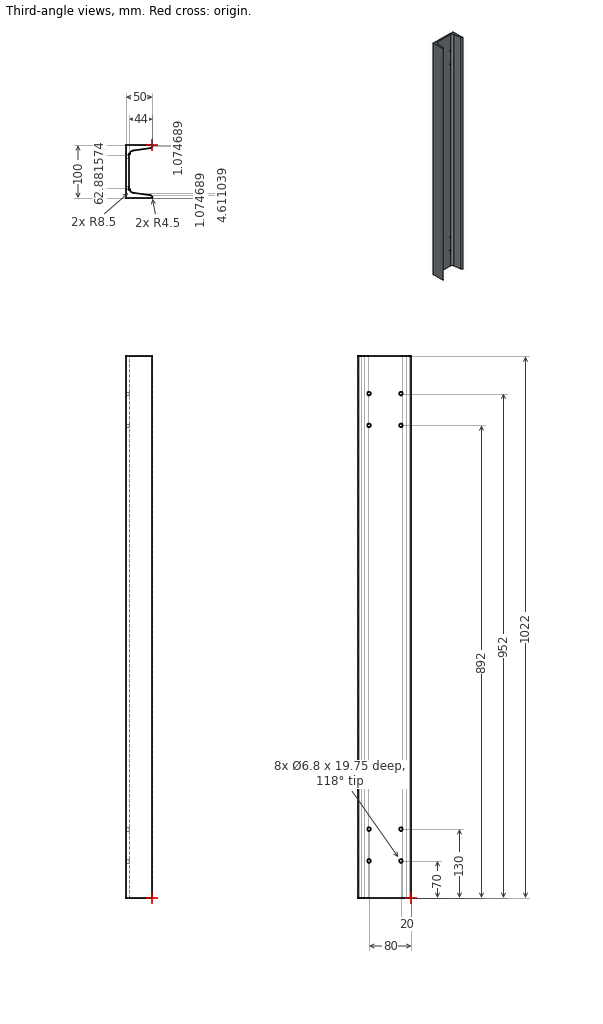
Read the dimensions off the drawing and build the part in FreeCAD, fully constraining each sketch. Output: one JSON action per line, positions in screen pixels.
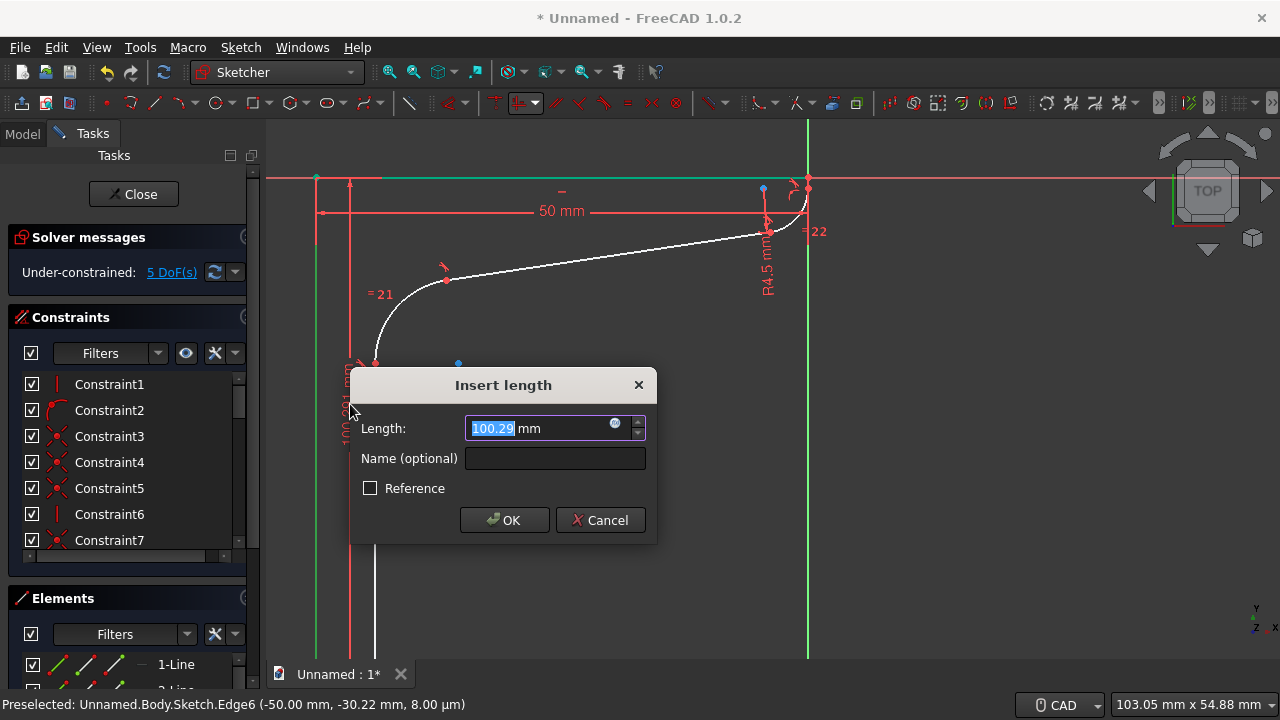
{"action": "type", "text": "100"}
{"action": "key", "text": "Return"}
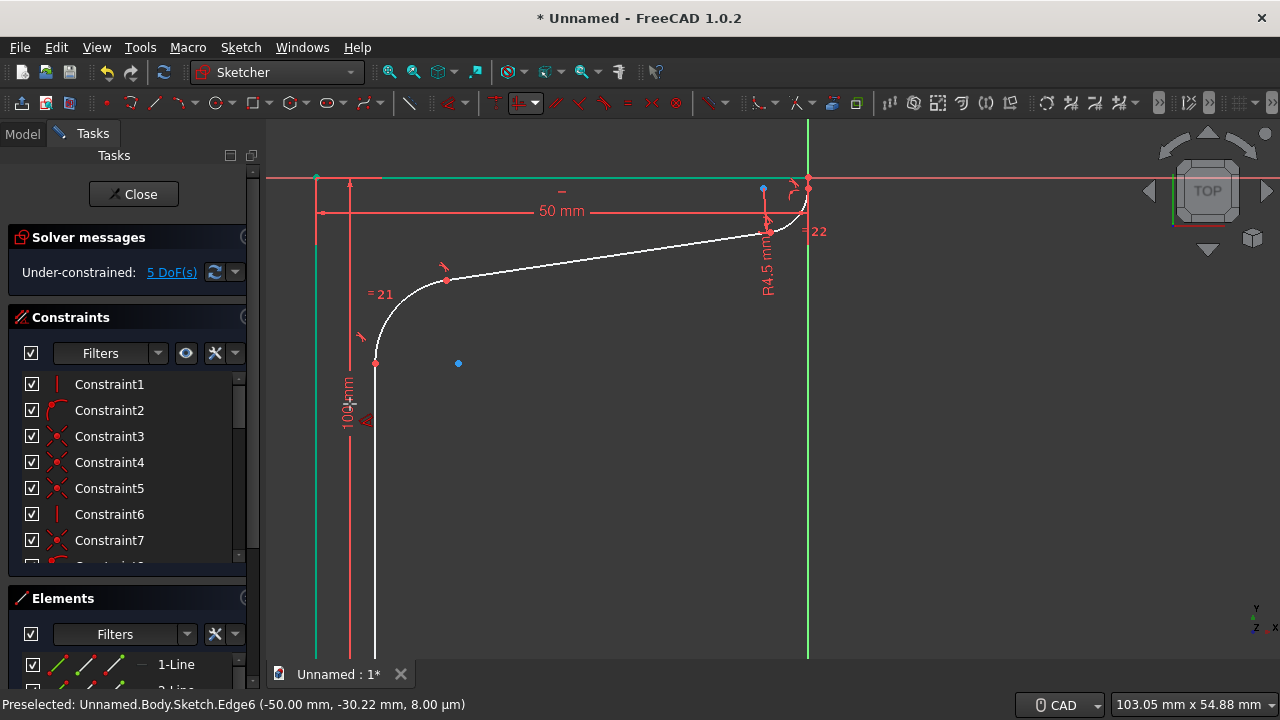
{"action": "scroll", "coordinate": [787, 226], "scroll_direction": "down", "scroll_amount": 5}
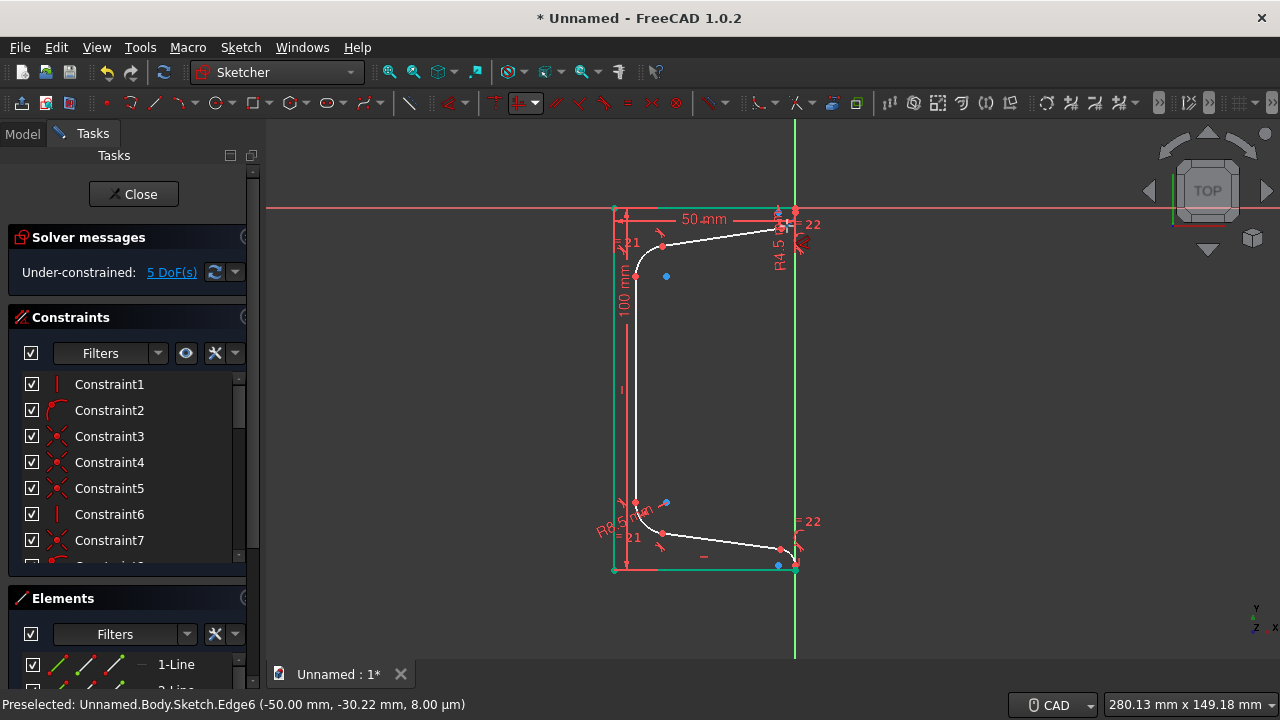
{"action": "left_click", "coordinate": [636, 503]}
{"action": "left_click", "coordinate": [715, 174]}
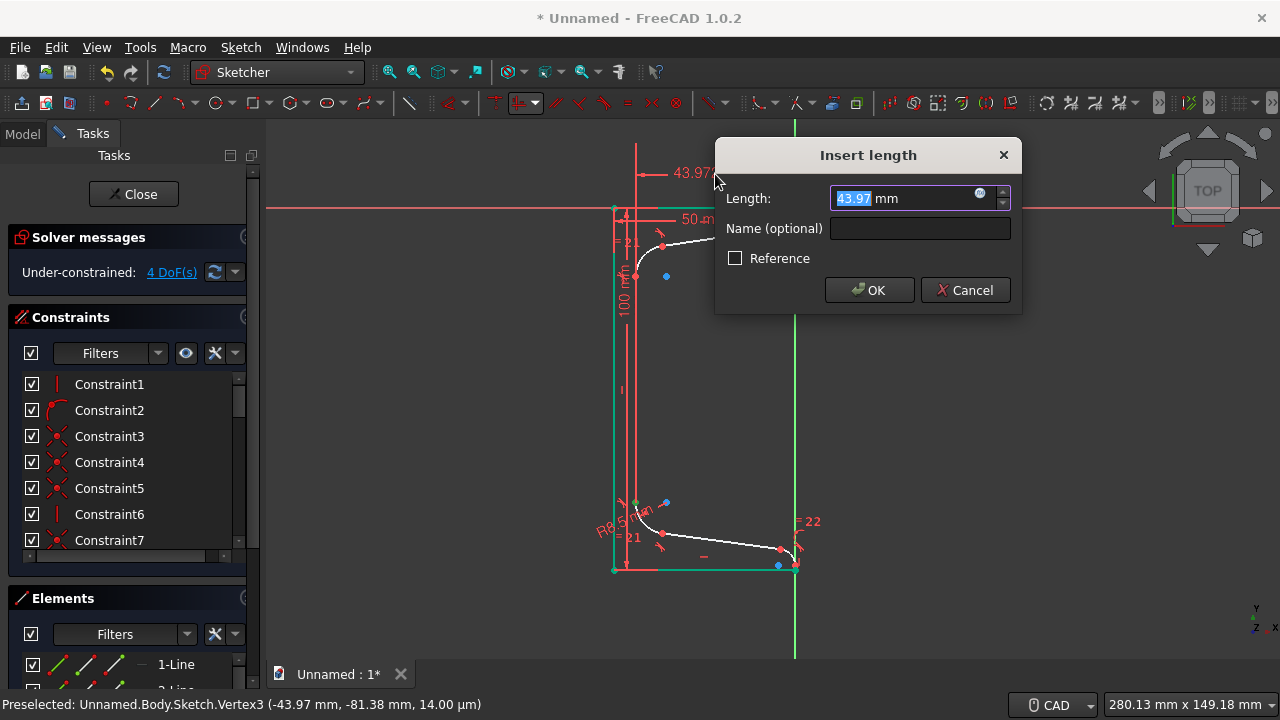
{"action": "type", "text": "44"}
{"action": "key", "text": "Return"}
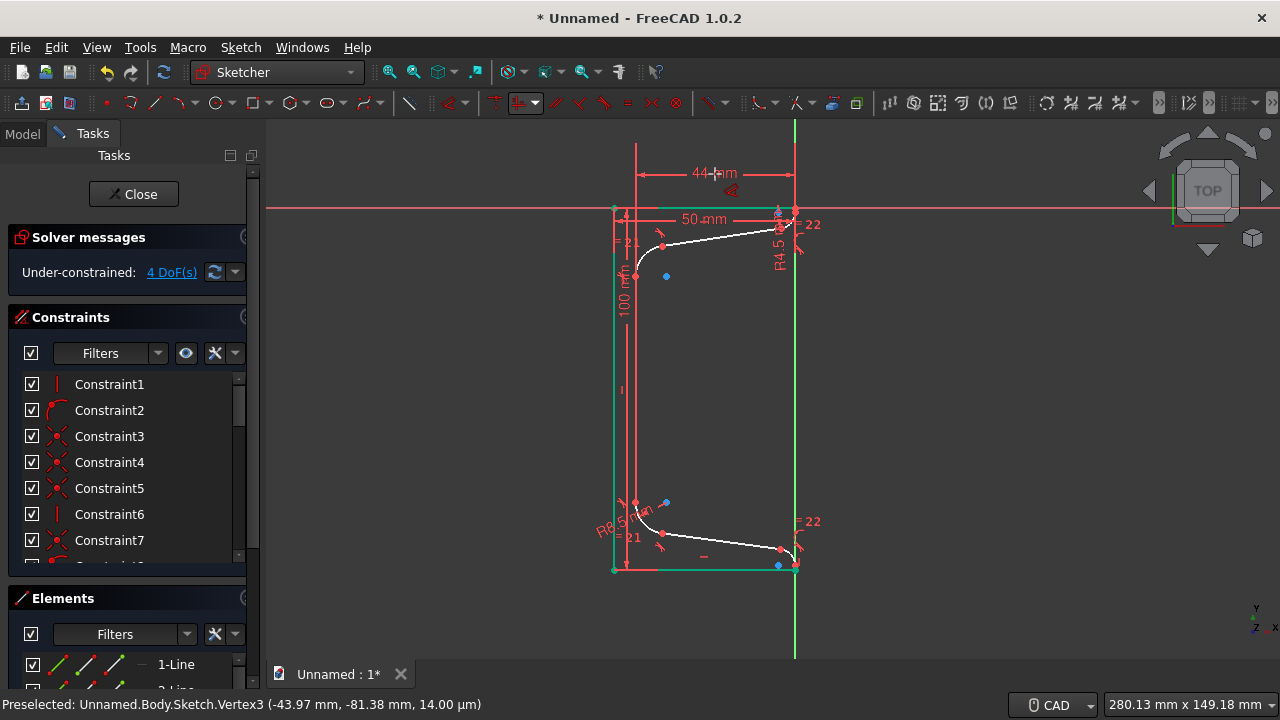
{"action": "scroll", "coordinate": [795, 210], "scroll_direction": "up", "scroll_amount": 12}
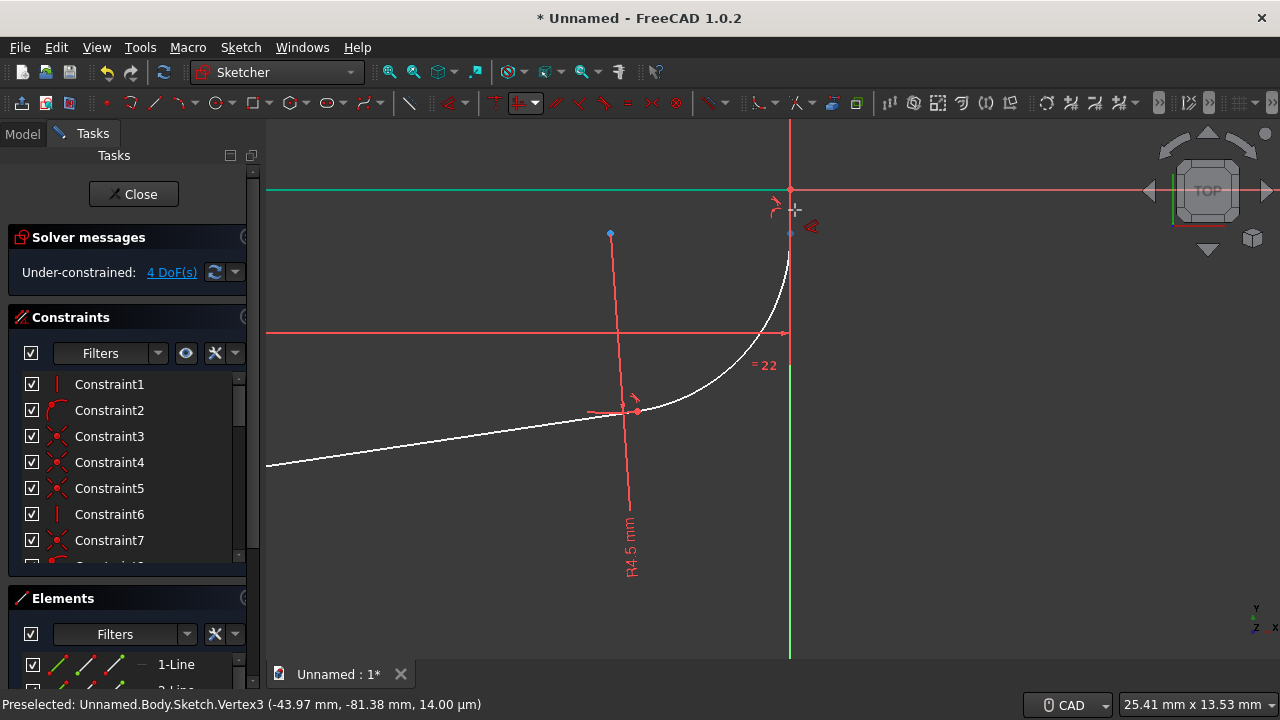
{"action": "left_click", "coordinate": [790, 212]}
{"action": "left_click", "coordinate": [824, 212]}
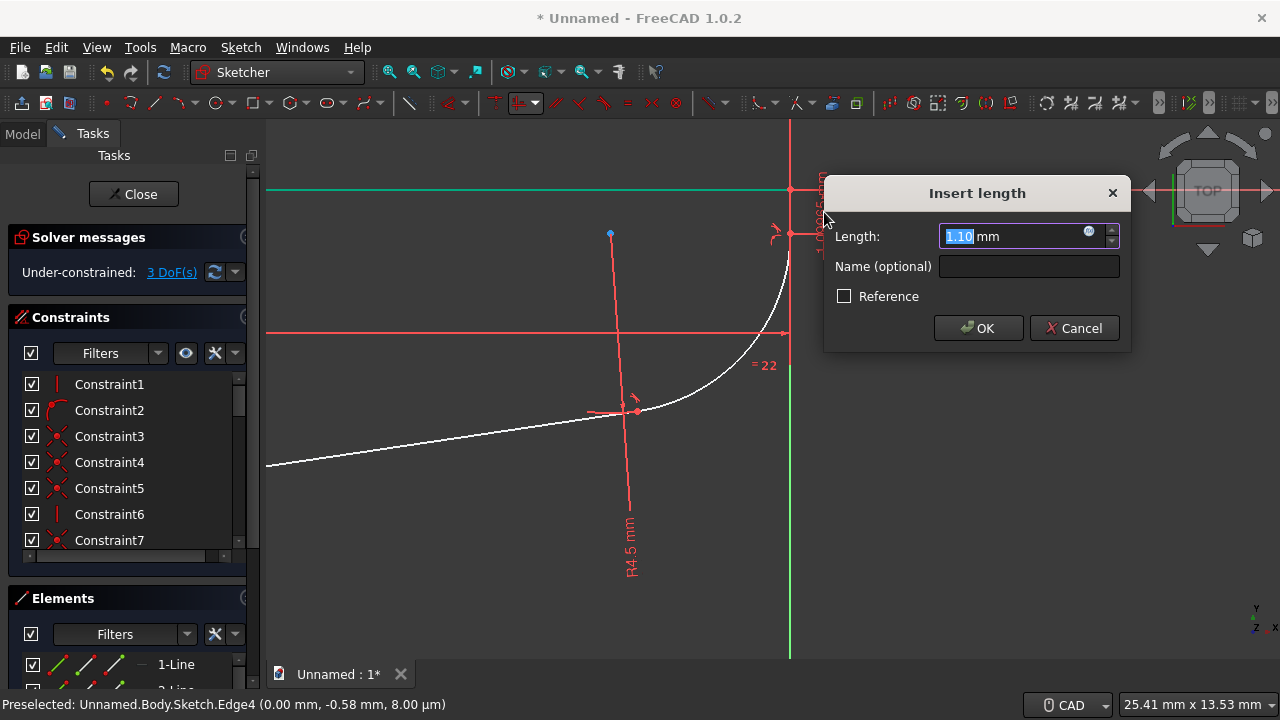
{"action": "type", "text": "1.074689"}
{"action": "key", "text": "Return"}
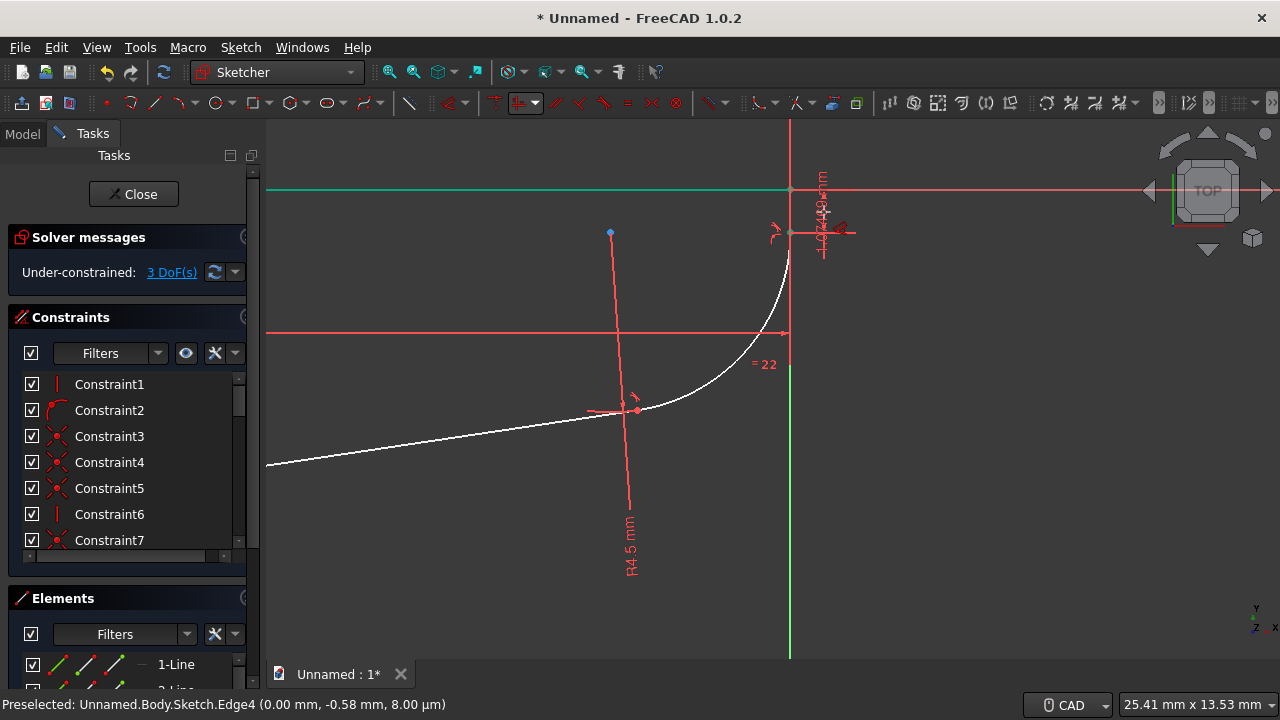
{"action": "scroll", "coordinate": [795, 210], "scroll_direction": "down", "scroll_amount": 12}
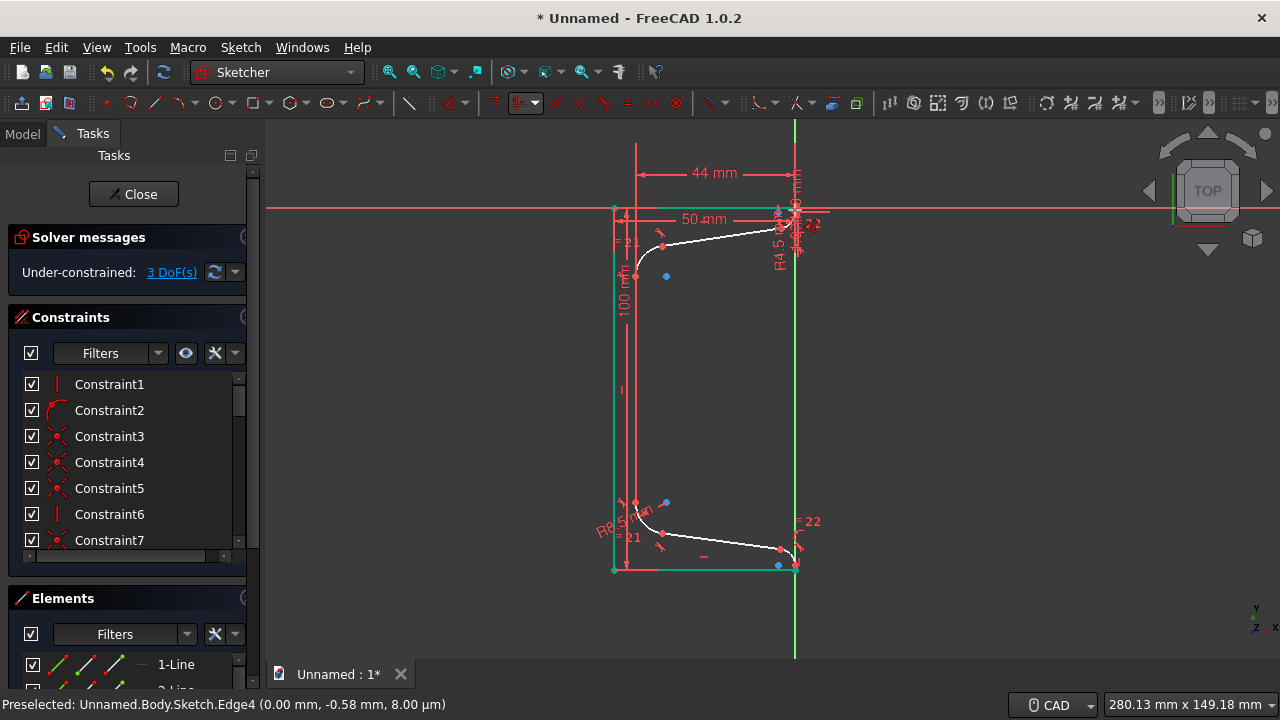
{"action": "scroll", "coordinate": [795, 569], "scroll_direction": "up", "scroll_amount": 12}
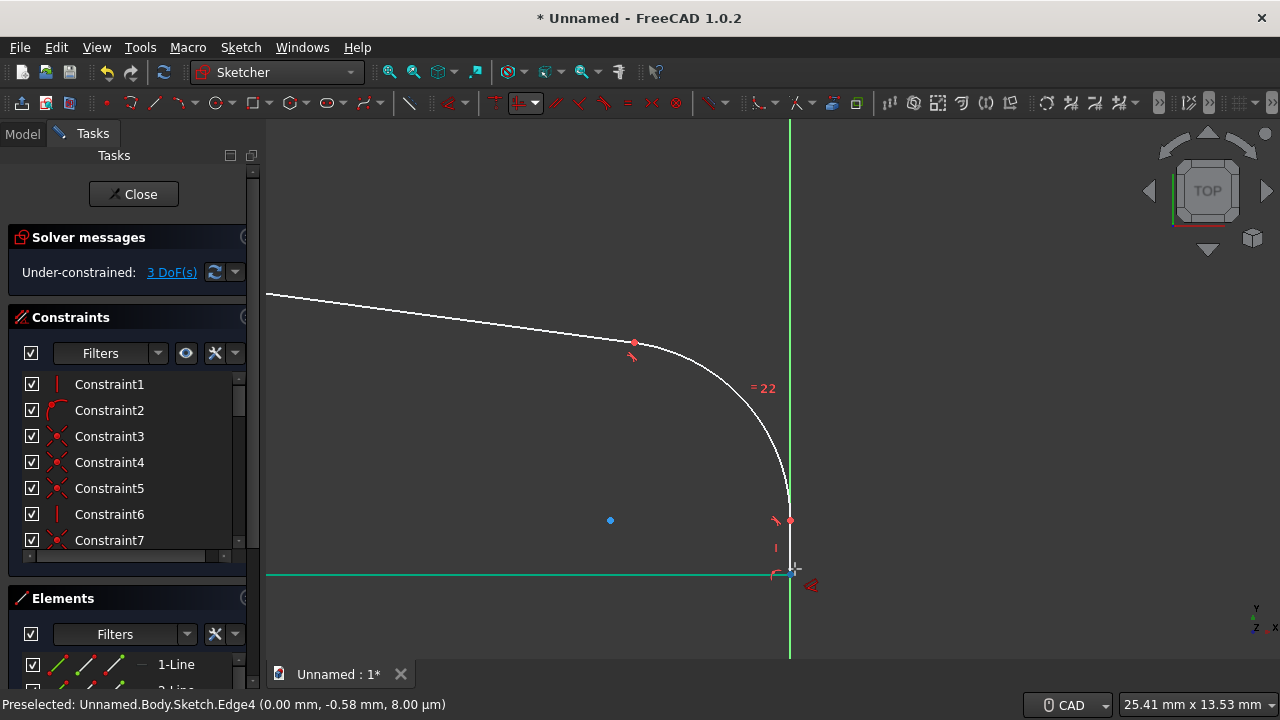
{"action": "left_click", "coordinate": [790, 559]}
{"action": "left_click", "coordinate": [824, 548]}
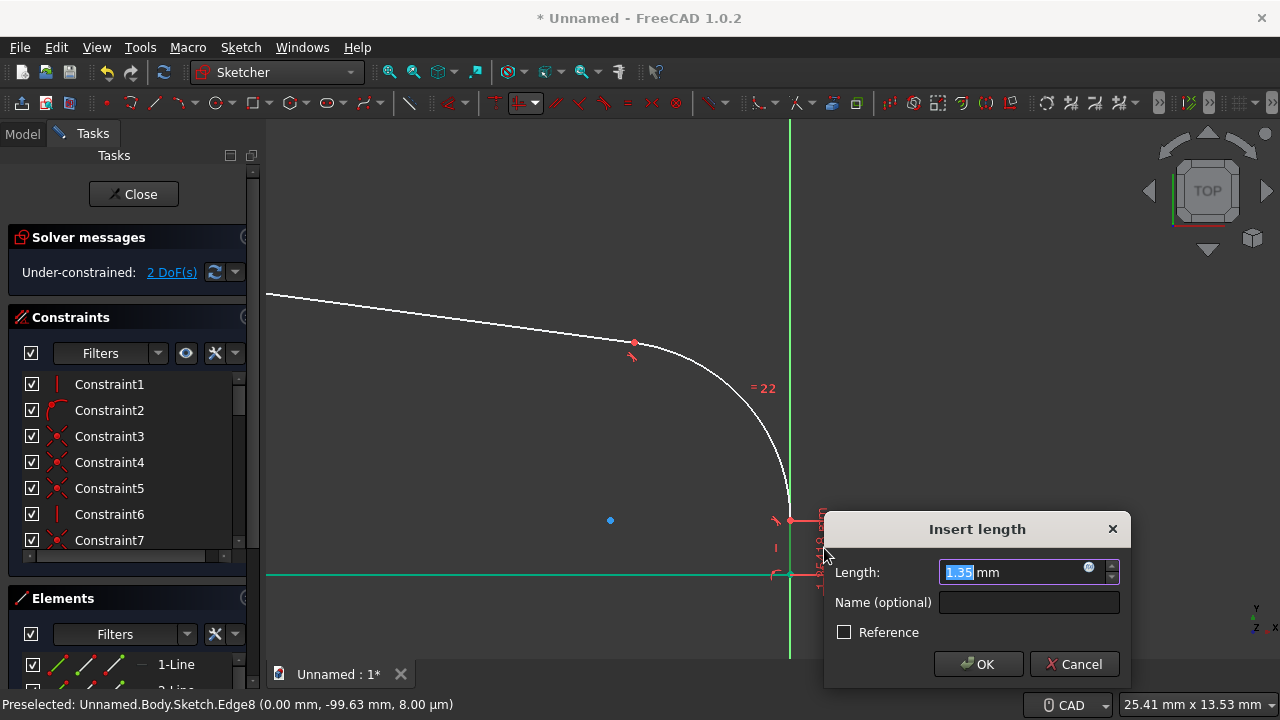
{"action": "type", "text": "1.074689"}
{"action": "key", "text": "Return"}